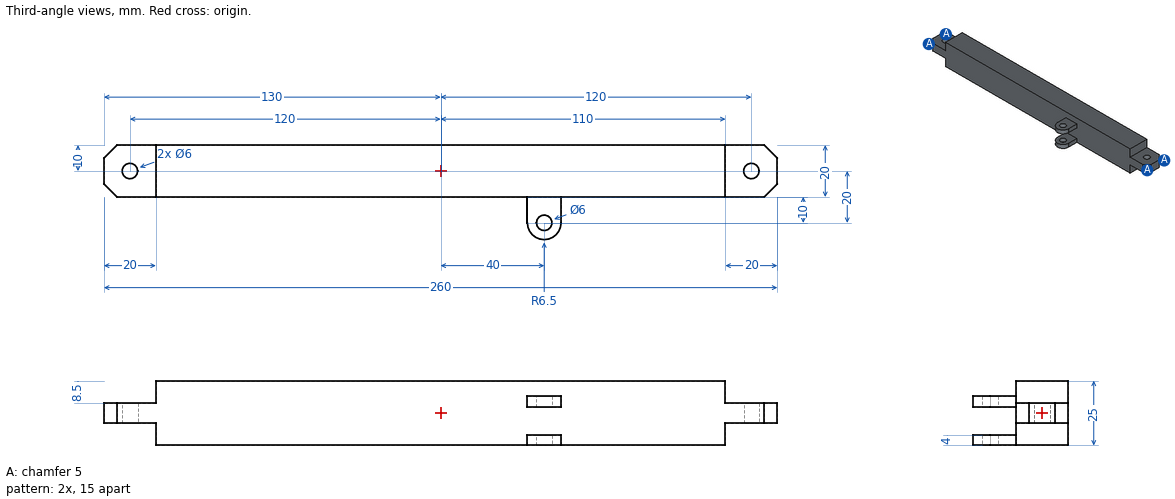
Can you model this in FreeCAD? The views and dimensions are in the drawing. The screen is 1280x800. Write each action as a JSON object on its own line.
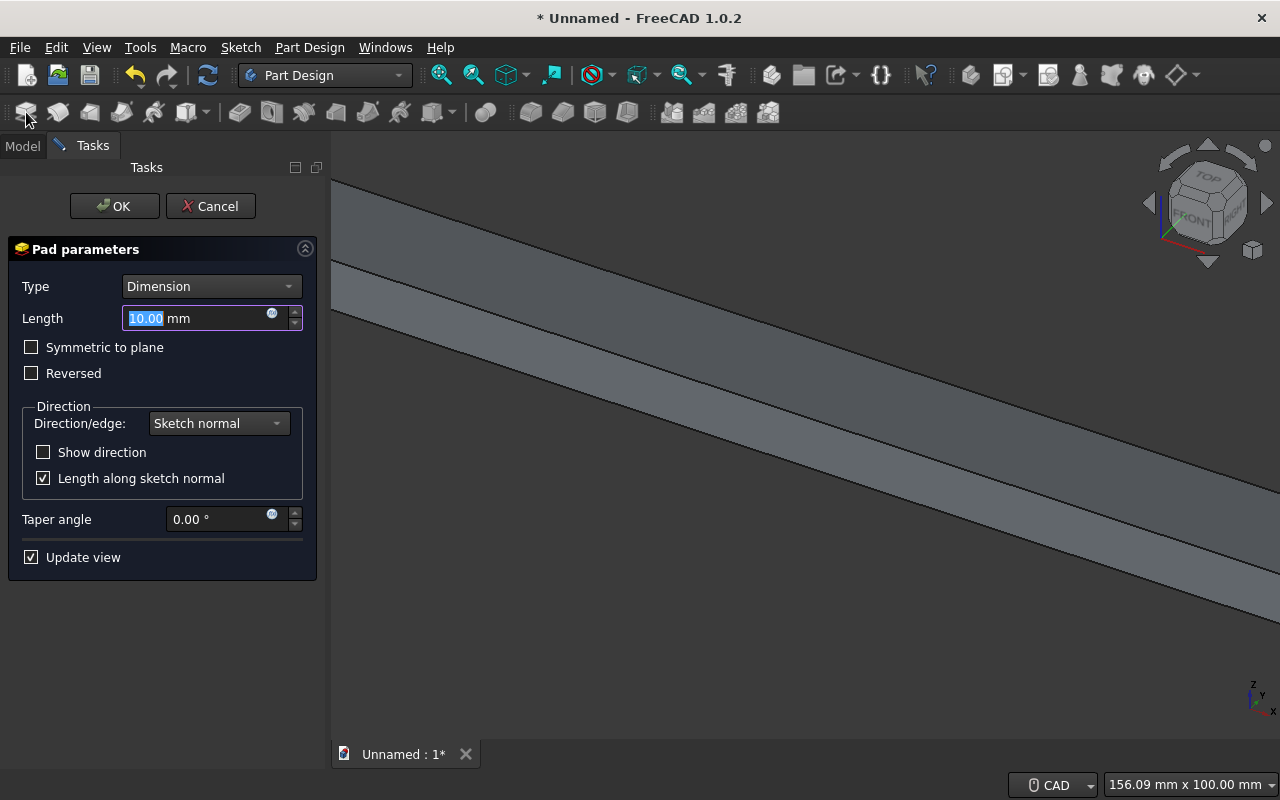
{"action": "type", "text": "25"}
{"action": "key", "text": "Tab"}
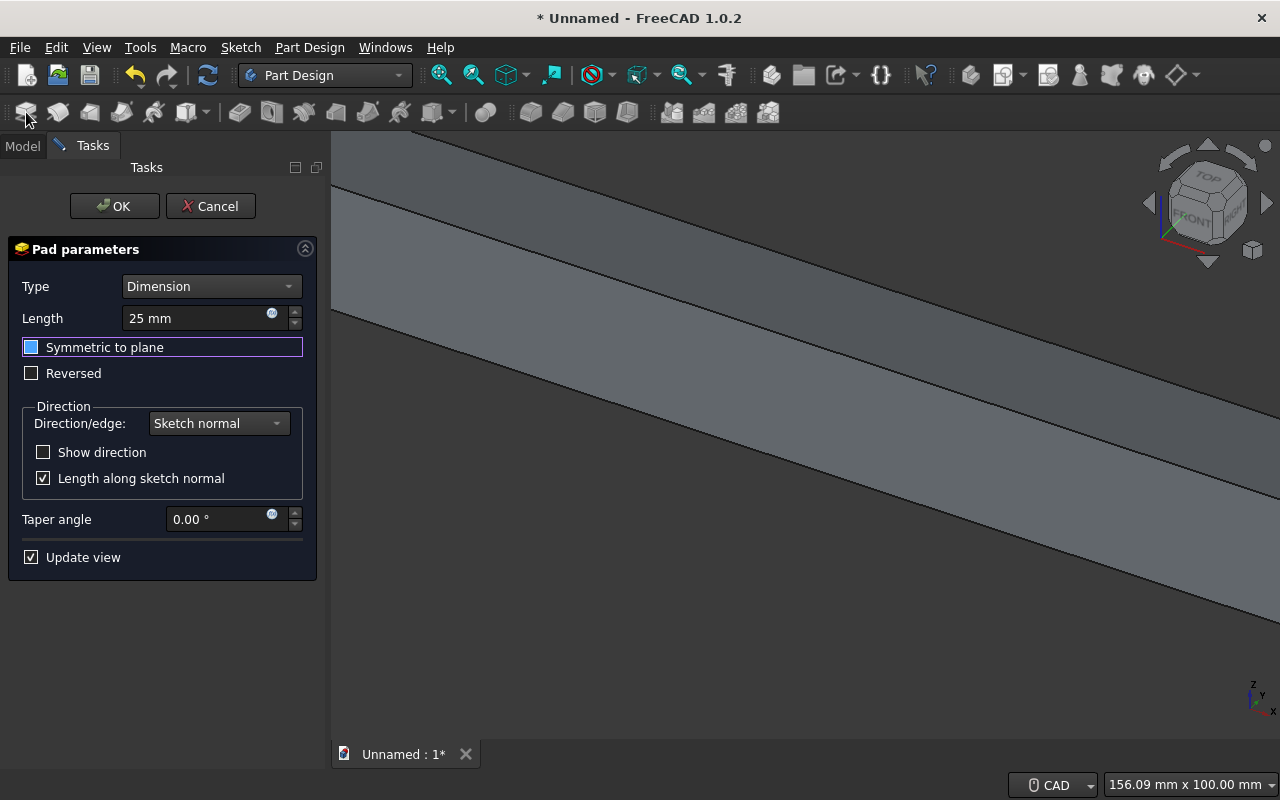
{"action": "left_click", "coordinate": [30, 347]}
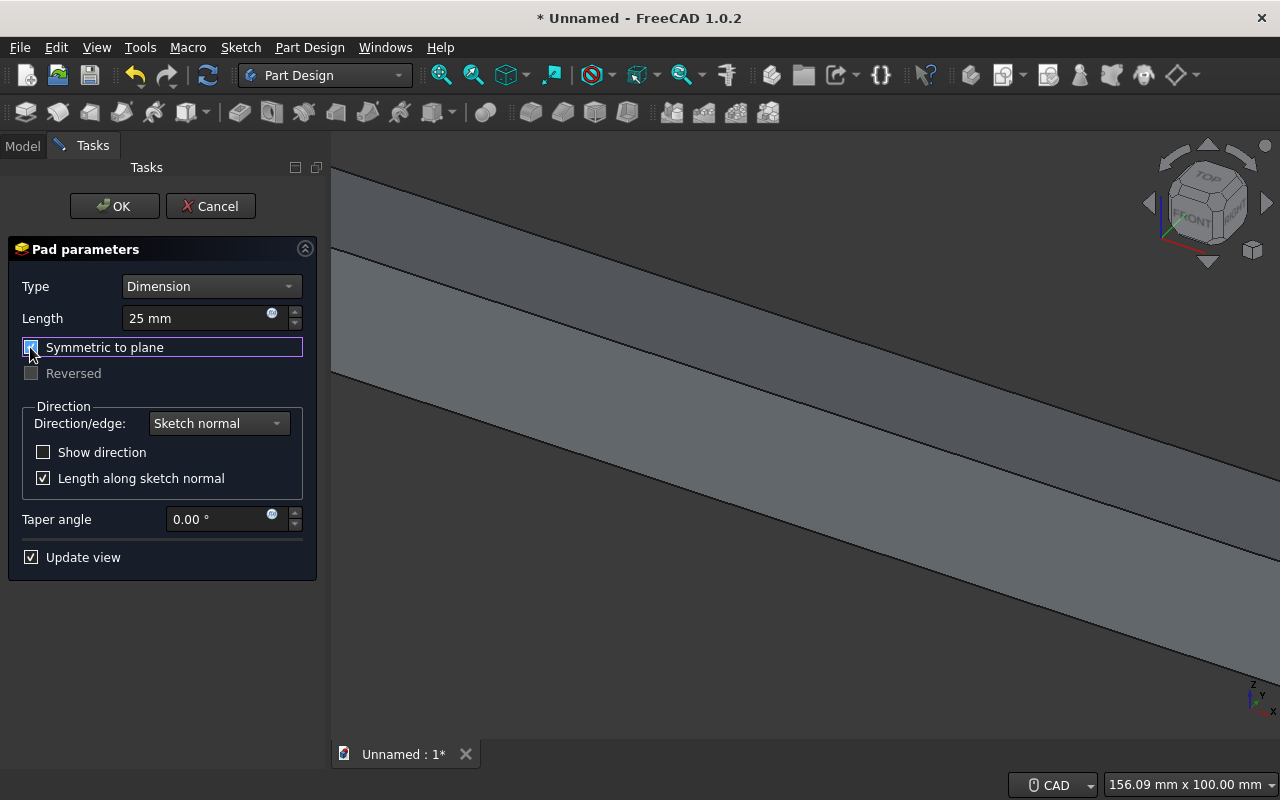
{"action": "left_click", "coordinate": [115, 206]}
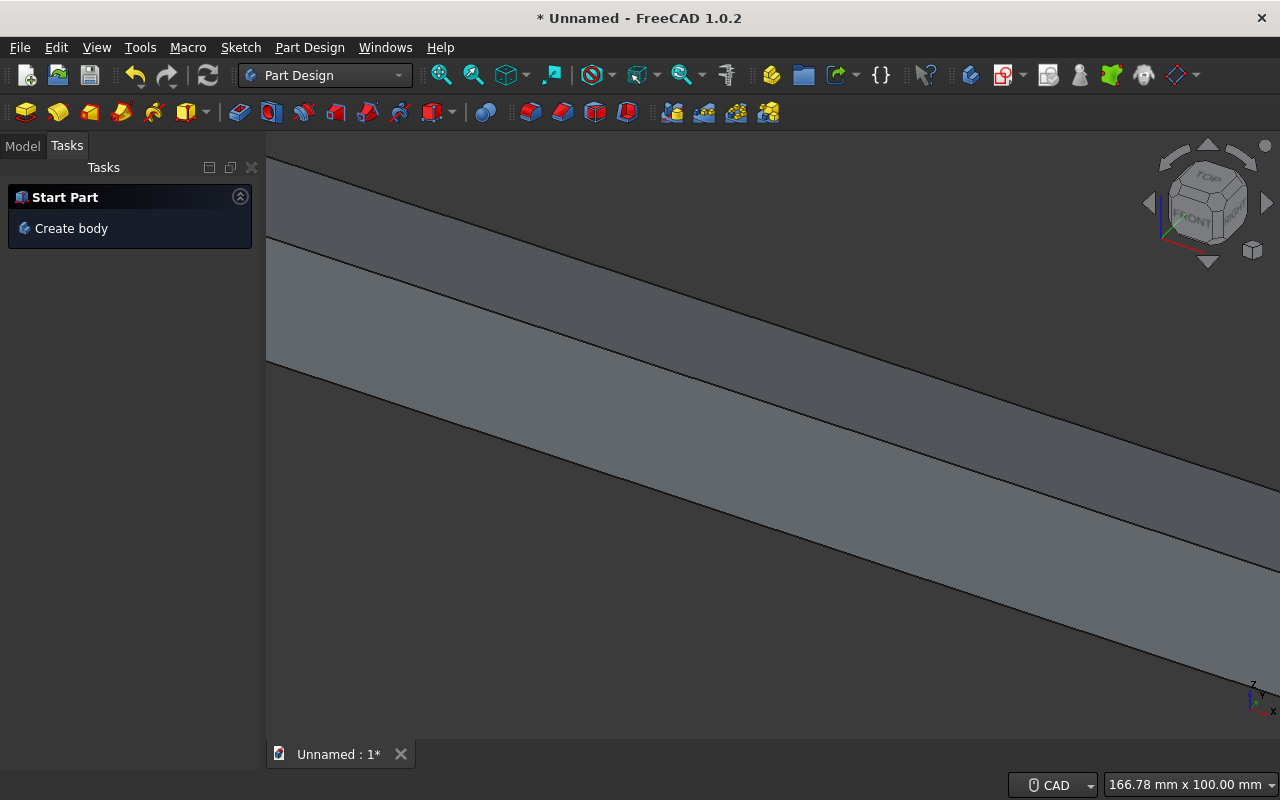
{"action": "left_click", "coordinate": [442, 76]}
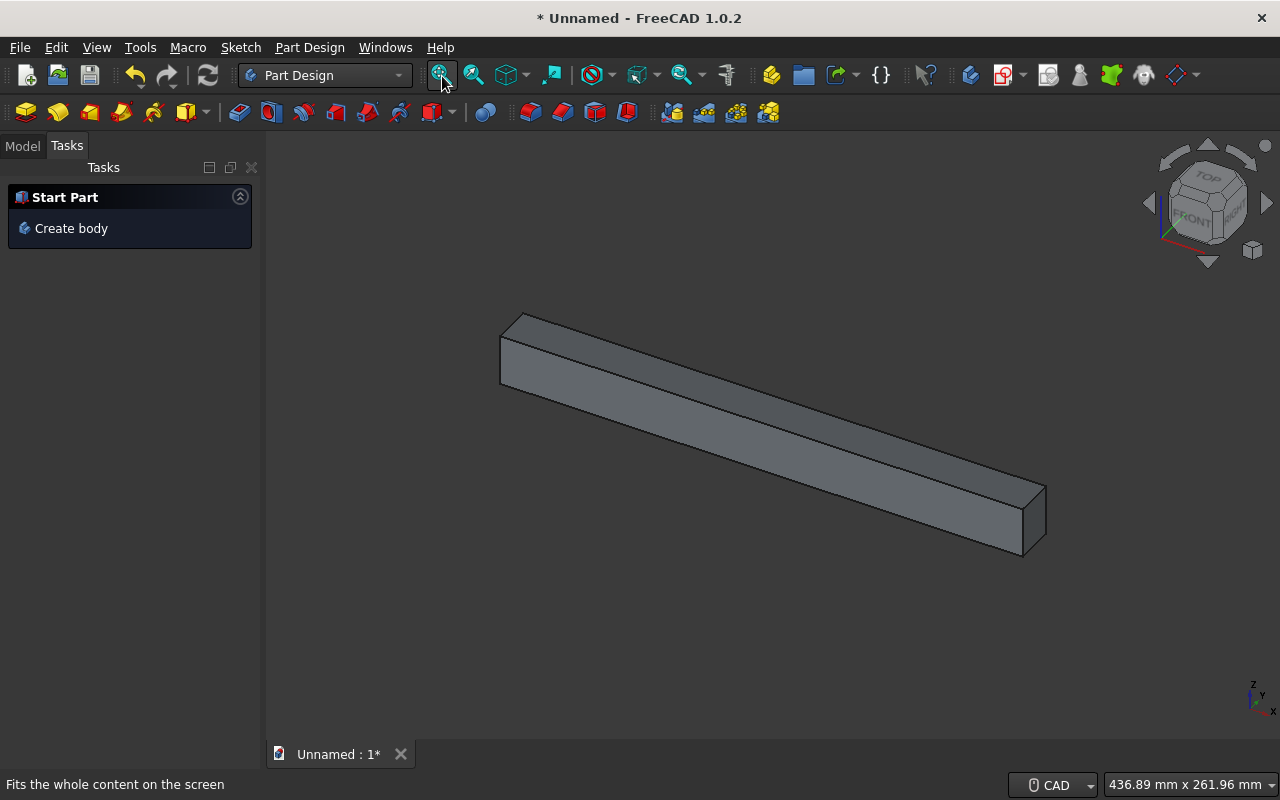
{"action": "left_click", "coordinate": [997, 484]}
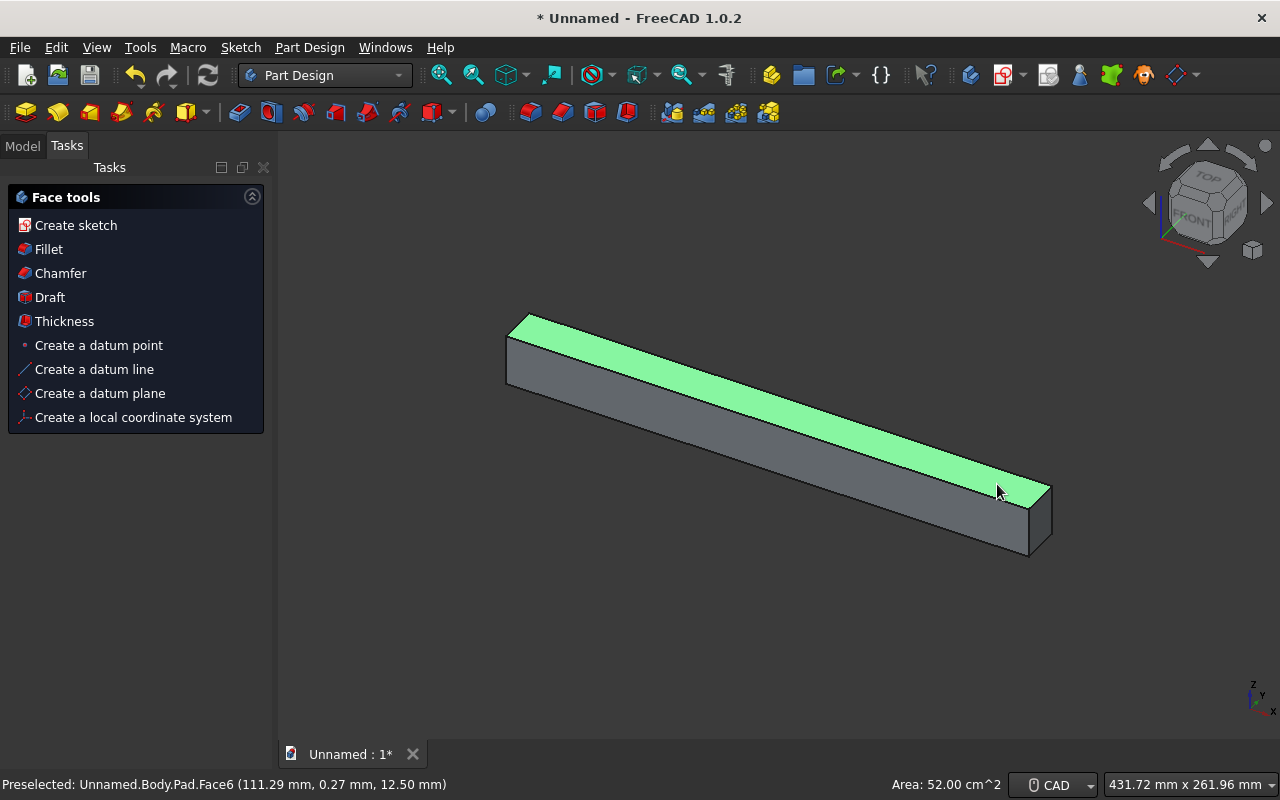
{"action": "left_click", "coordinate": [1004, 76]}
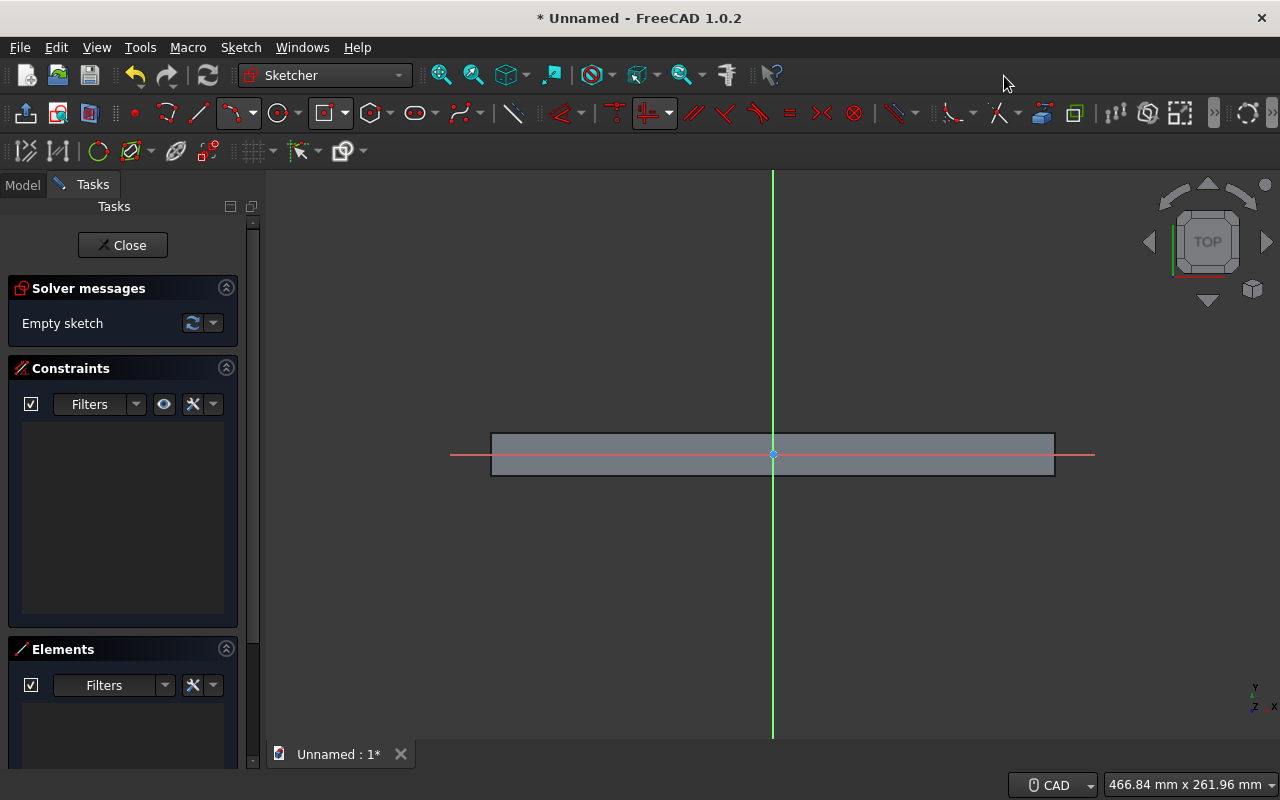
{"action": "key", "text": "g c"}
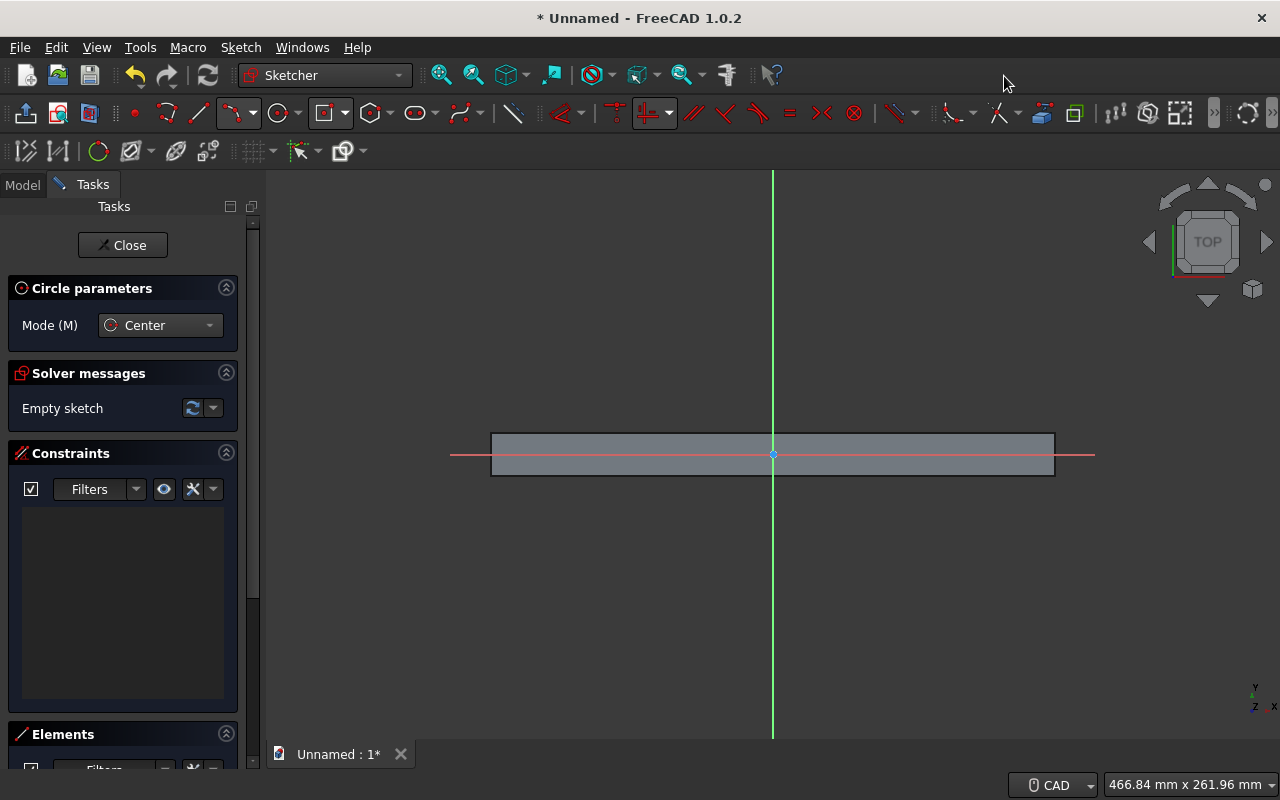
{"action": "scroll", "coordinate": [512, 454], "scroll_direction": "up", "scroll_amount": 7}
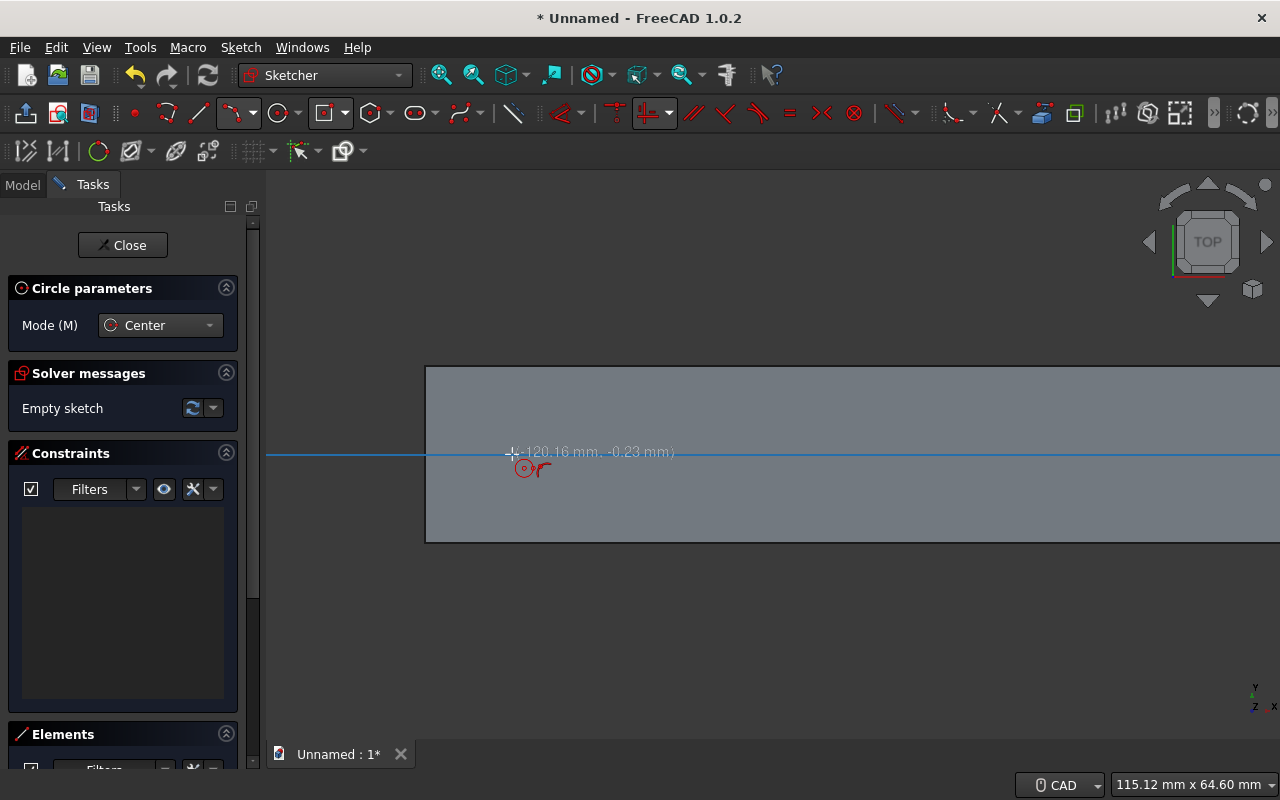
{"action": "scroll", "coordinate": [421, 454], "scroll_direction": "down", "scroll_amount": 7}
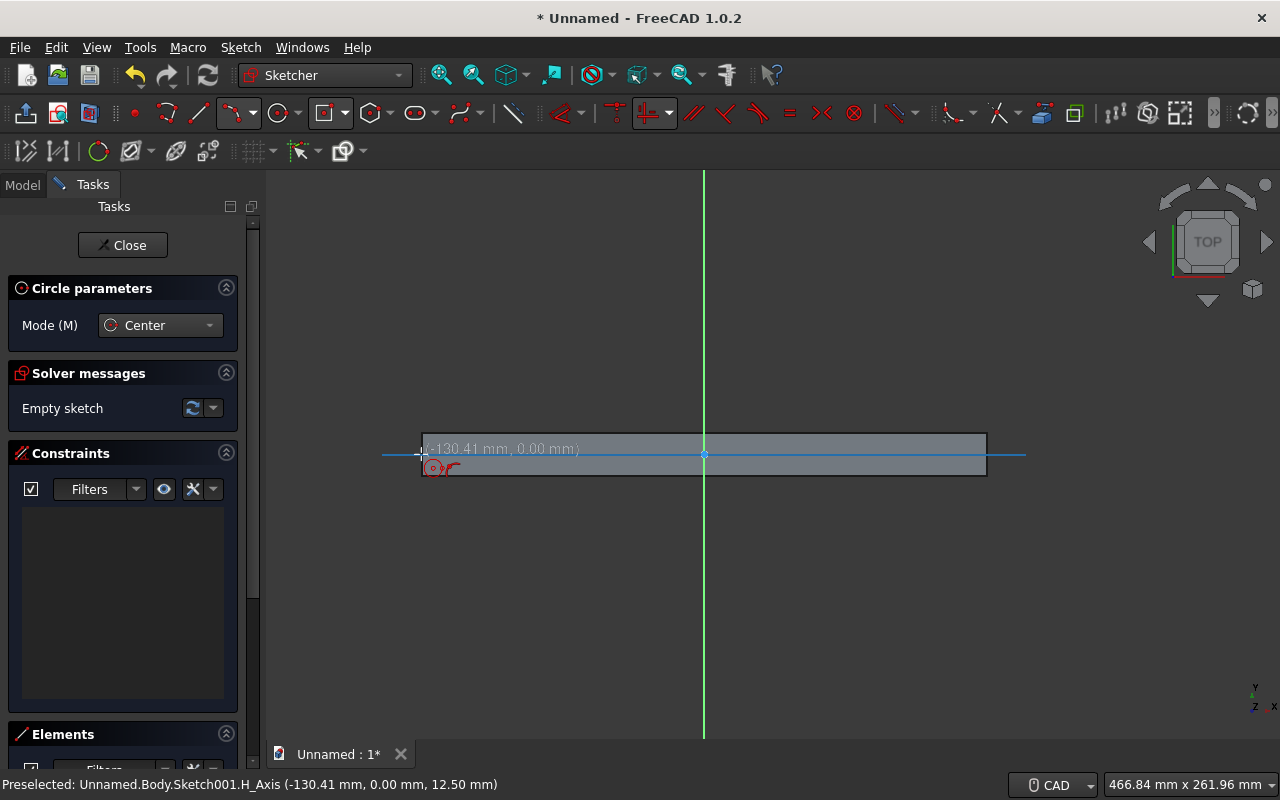
{"action": "left_click", "coordinate": [444, 454]}